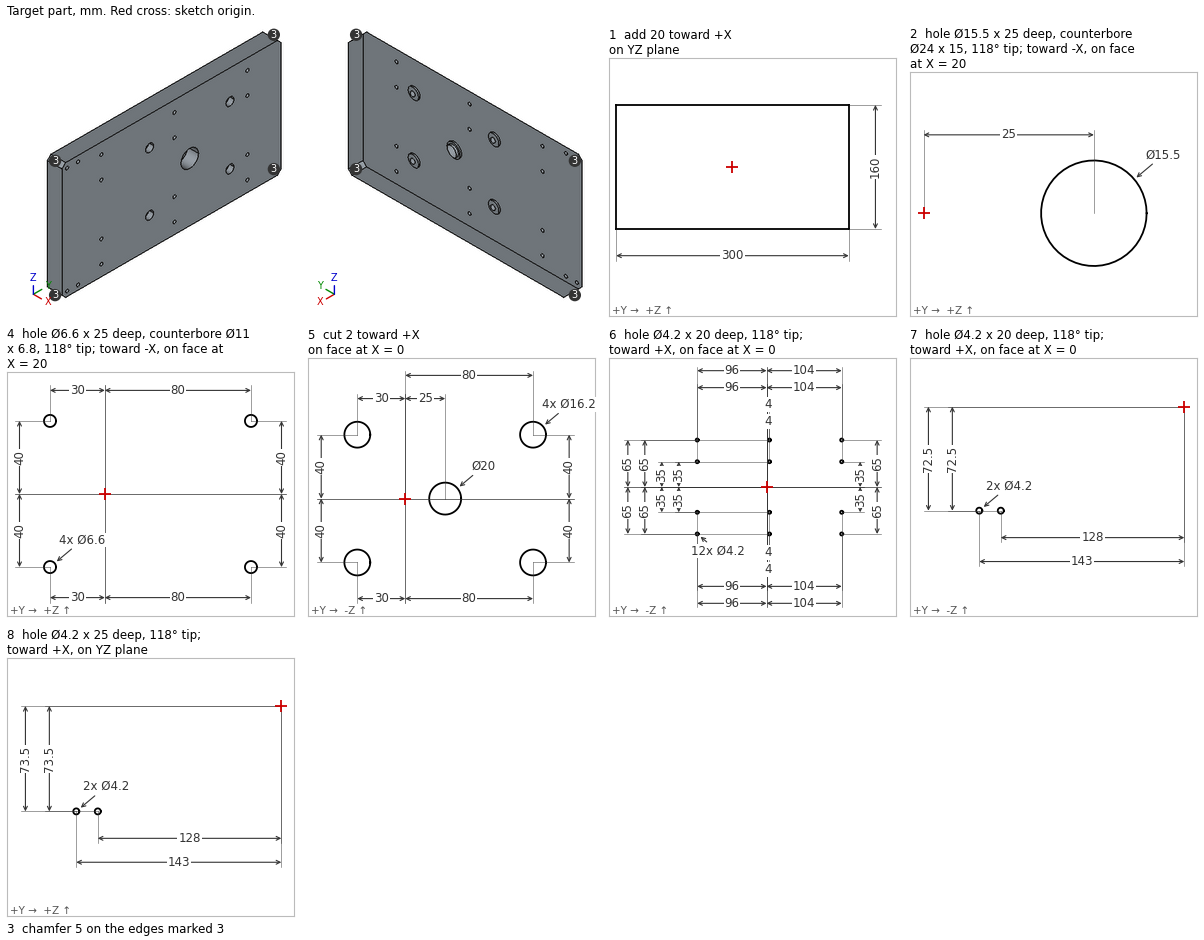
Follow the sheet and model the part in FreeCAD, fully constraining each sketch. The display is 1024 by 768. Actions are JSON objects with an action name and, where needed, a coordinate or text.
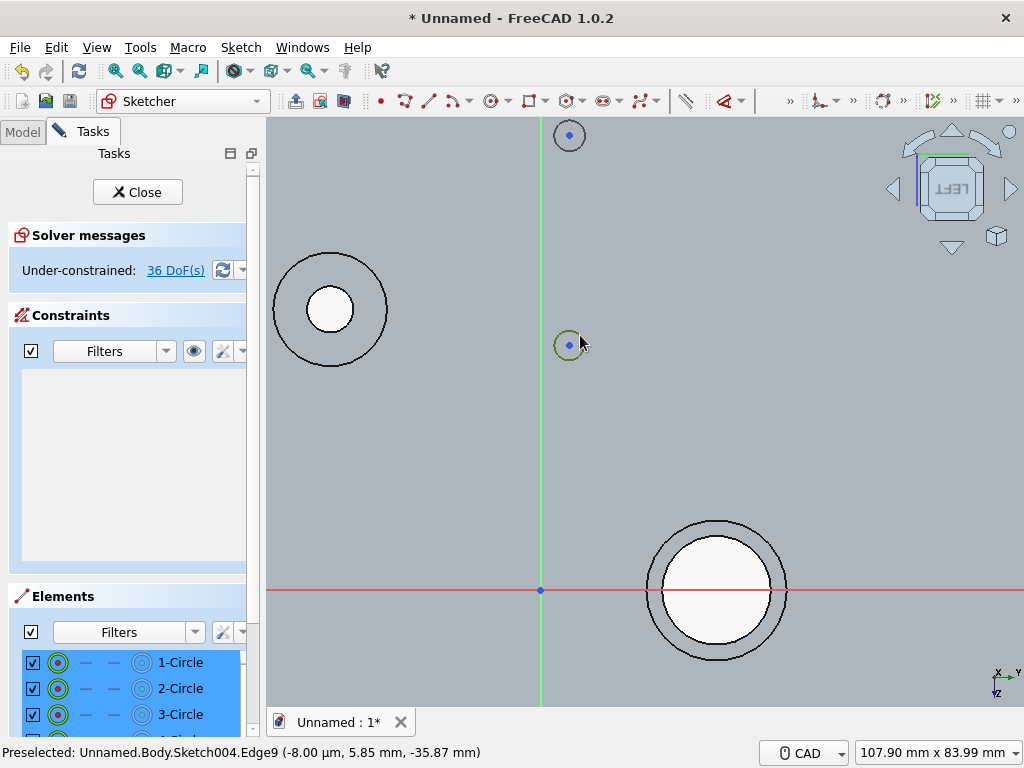
{"action": "left_click", "coordinate": [559, 147]}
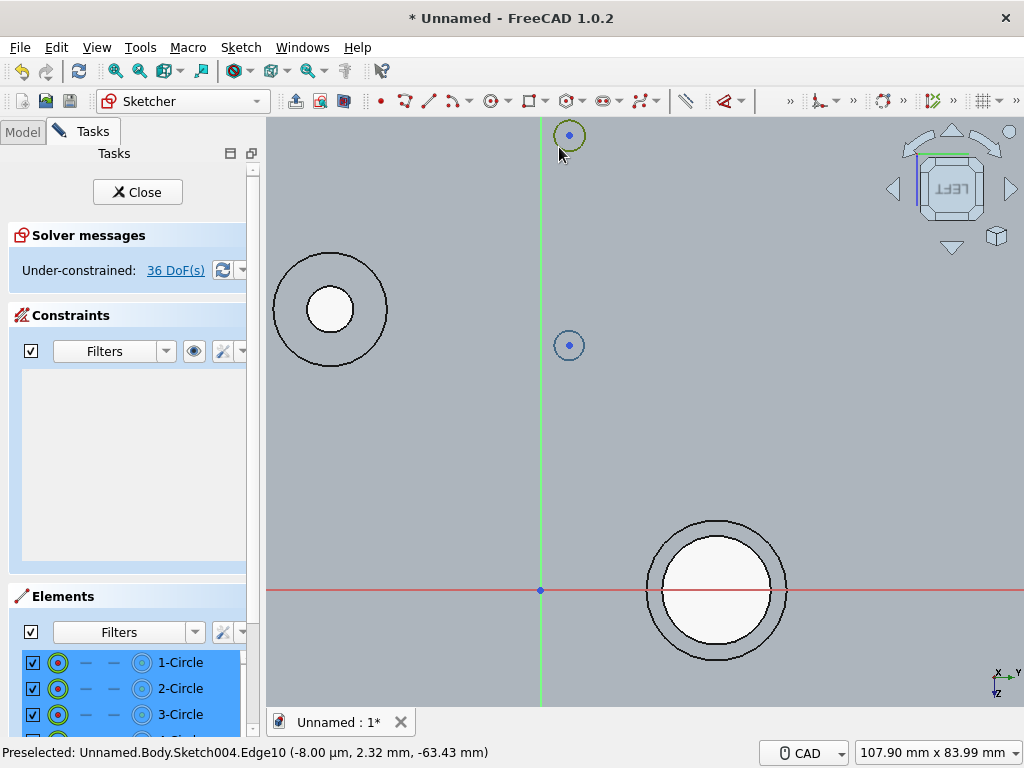
{"action": "scroll", "coordinate": [580, 335], "scroll_direction": "down", "scroll_amount": 6}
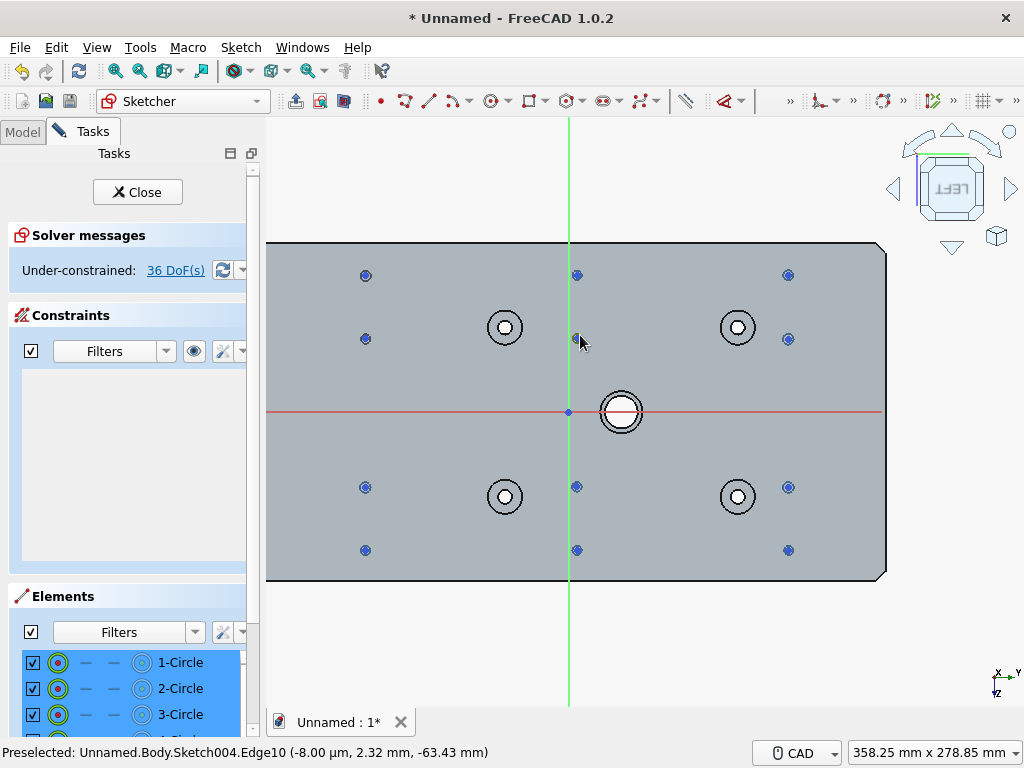
{"action": "scroll", "coordinate": [369, 336], "scroll_direction": "up", "scroll_amount": 6}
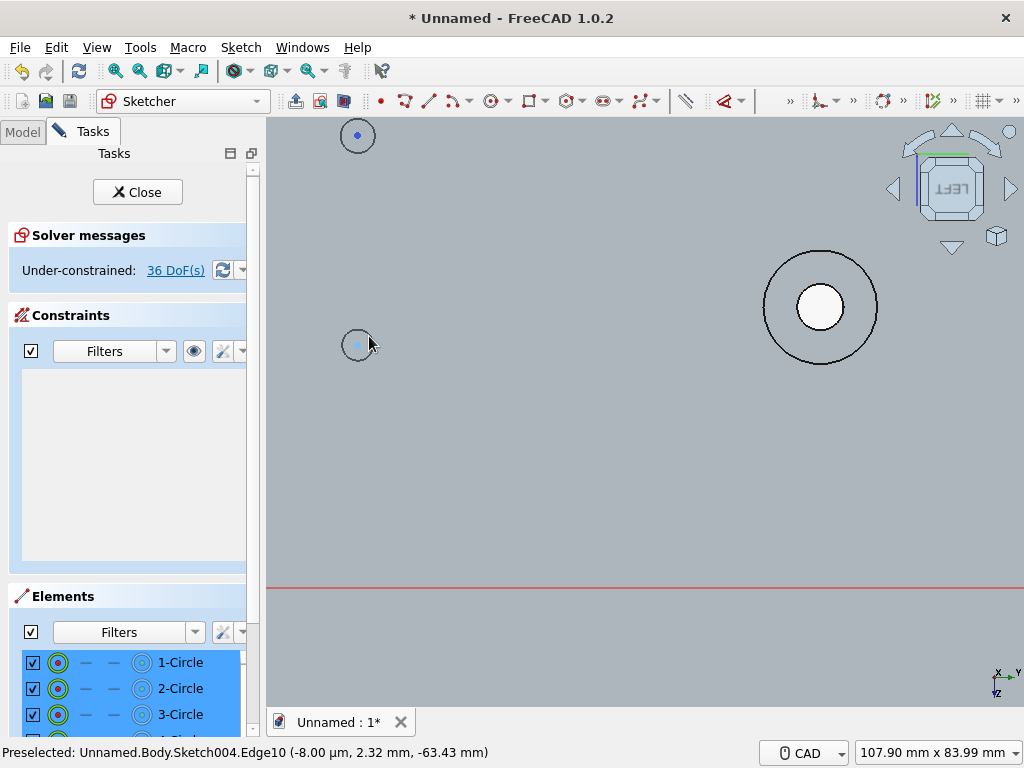
{"action": "left_click", "coordinate": [369, 334]}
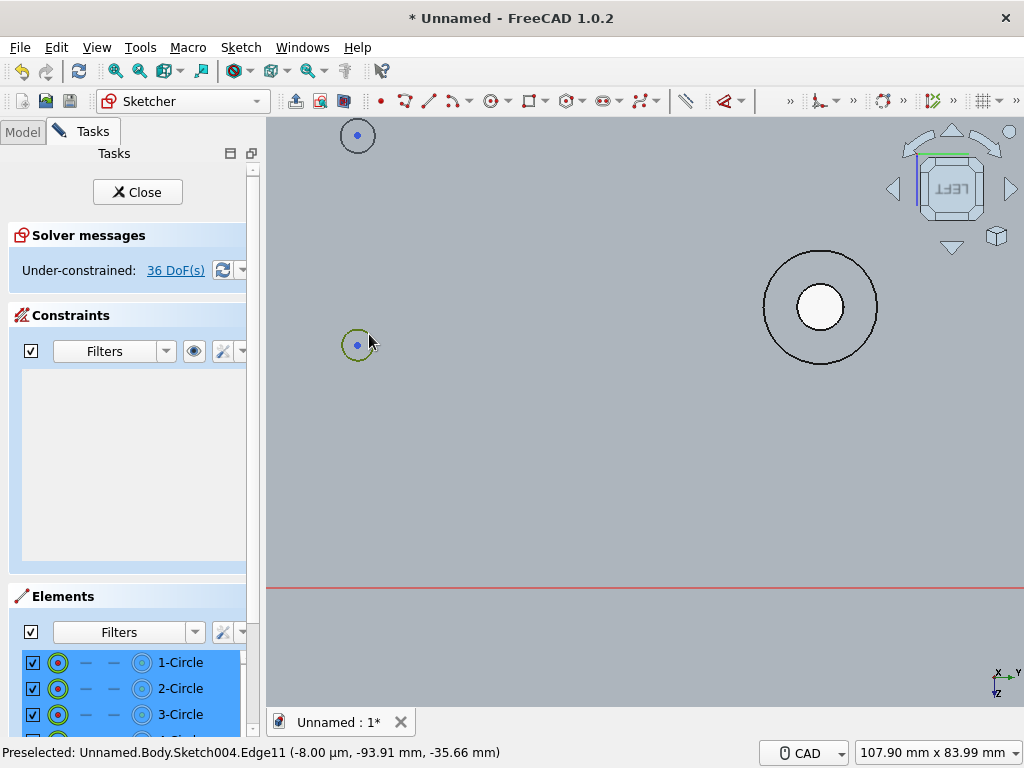
{"action": "left_click", "coordinate": [346, 148]}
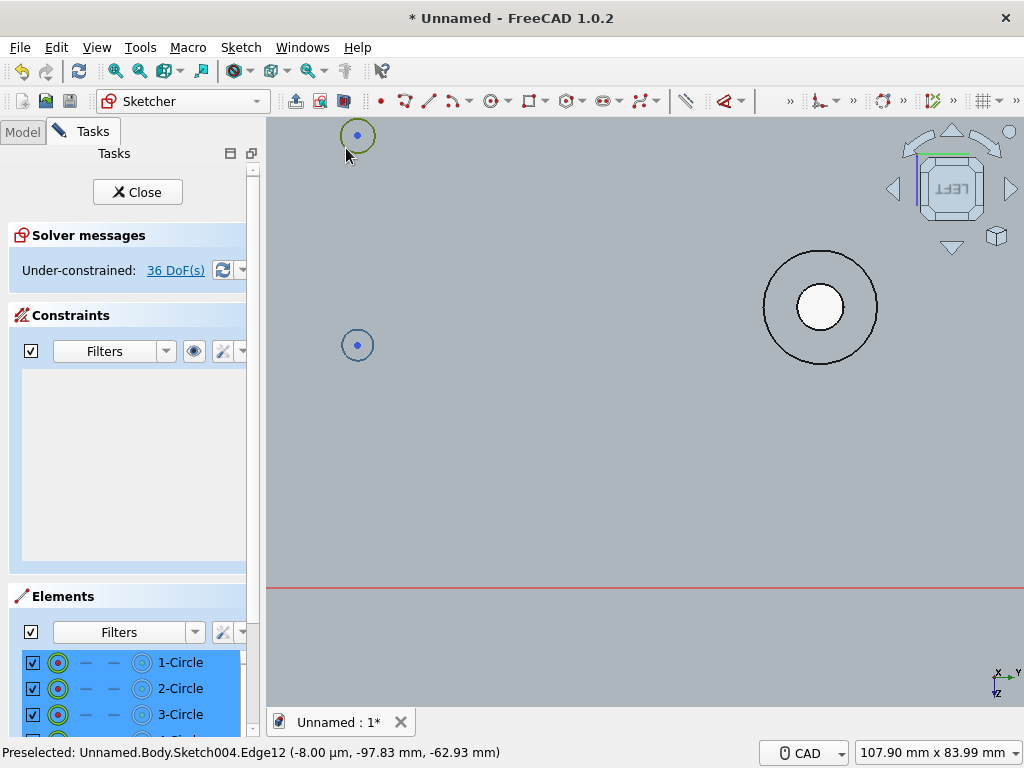
{"action": "key", "text": "e"}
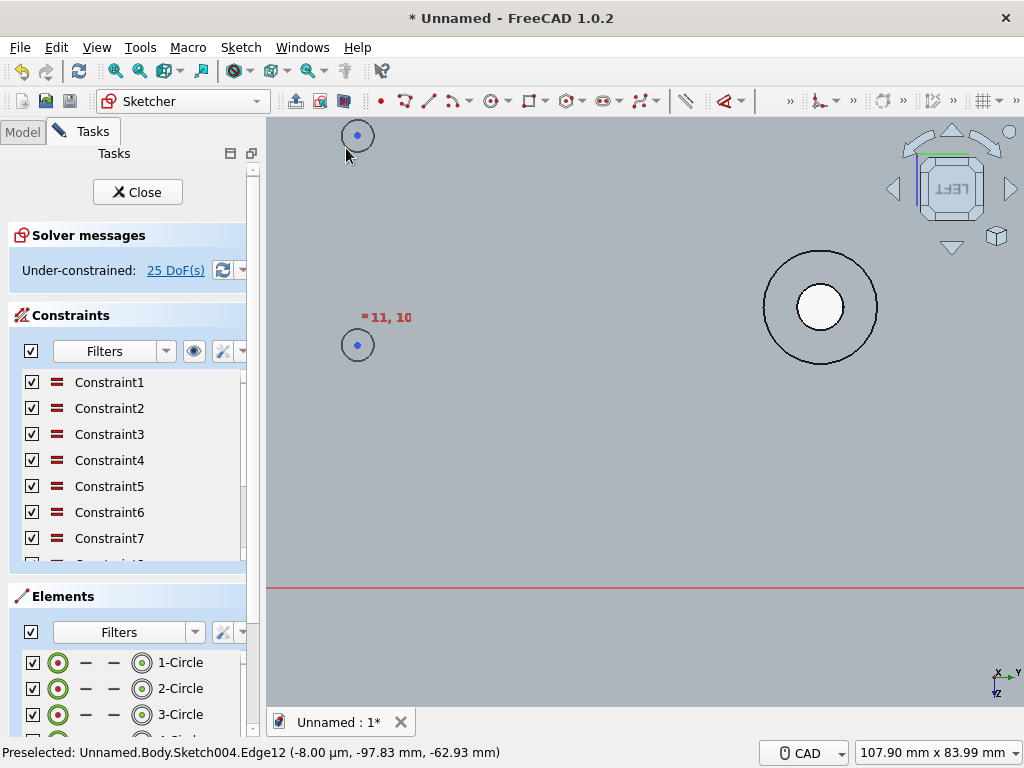
{"action": "key", "text": "d"}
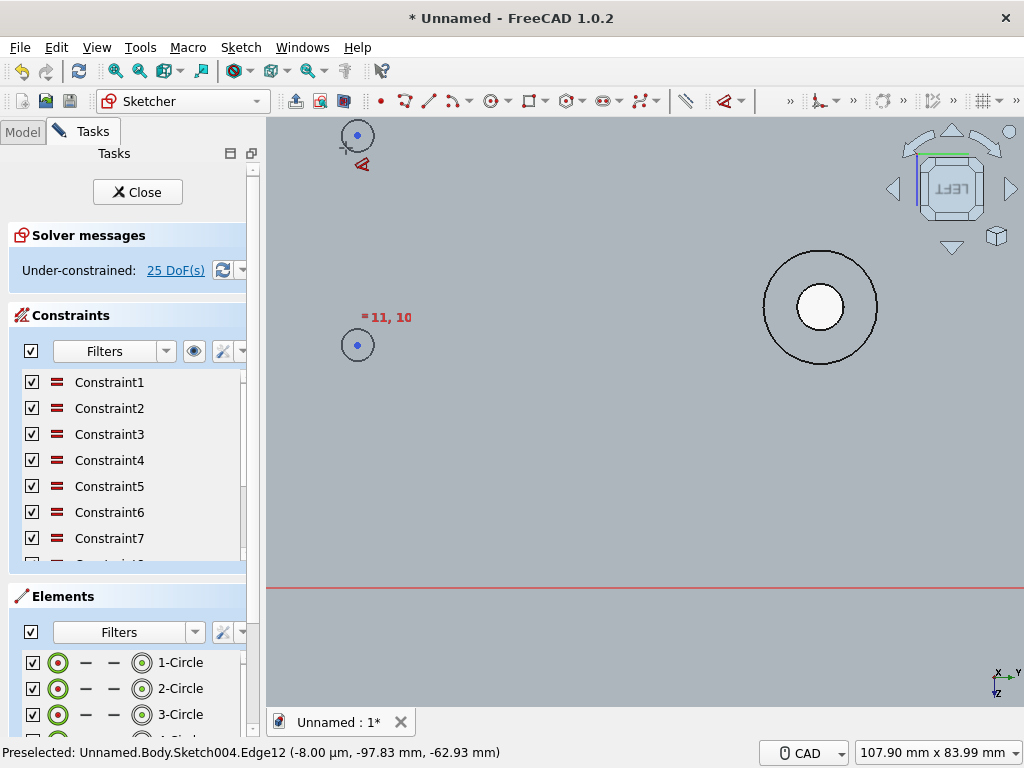
{"action": "scroll", "coordinate": [368, 336], "scroll_direction": "down", "scroll_amount": 6}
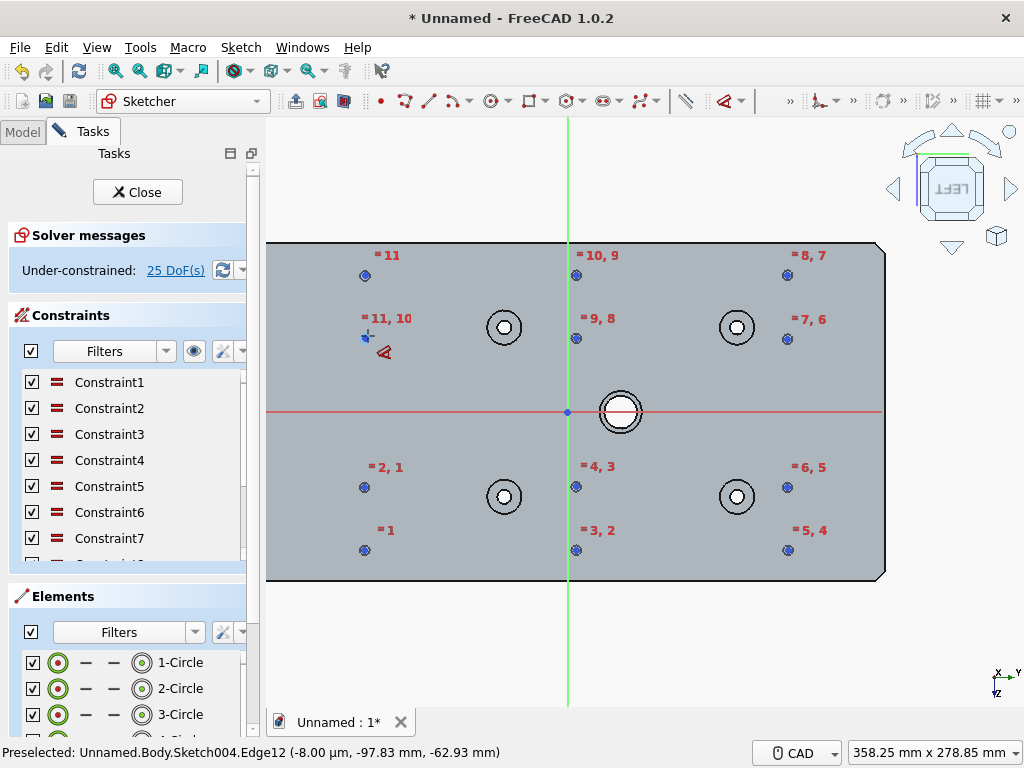
{"action": "scroll", "coordinate": [368, 547], "scroll_direction": "up", "scroll_amount": 8}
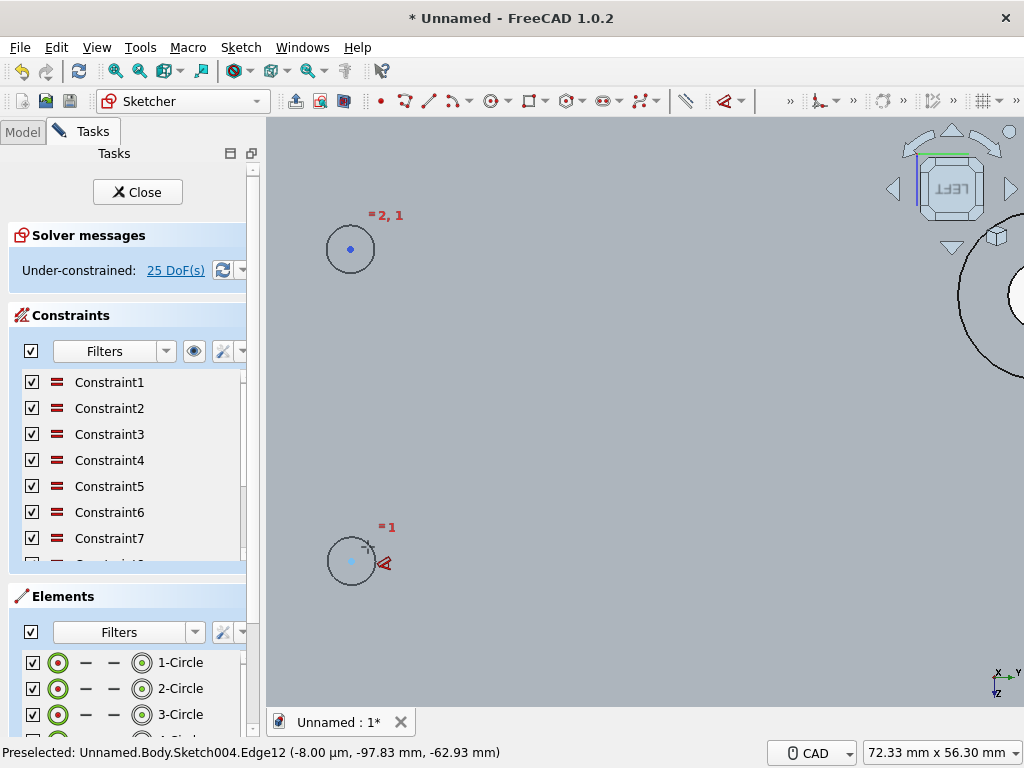
{"action": "left_click", "coordinate": [368, 544]}
{"action": "left_click", "coordinate": [390, 521]}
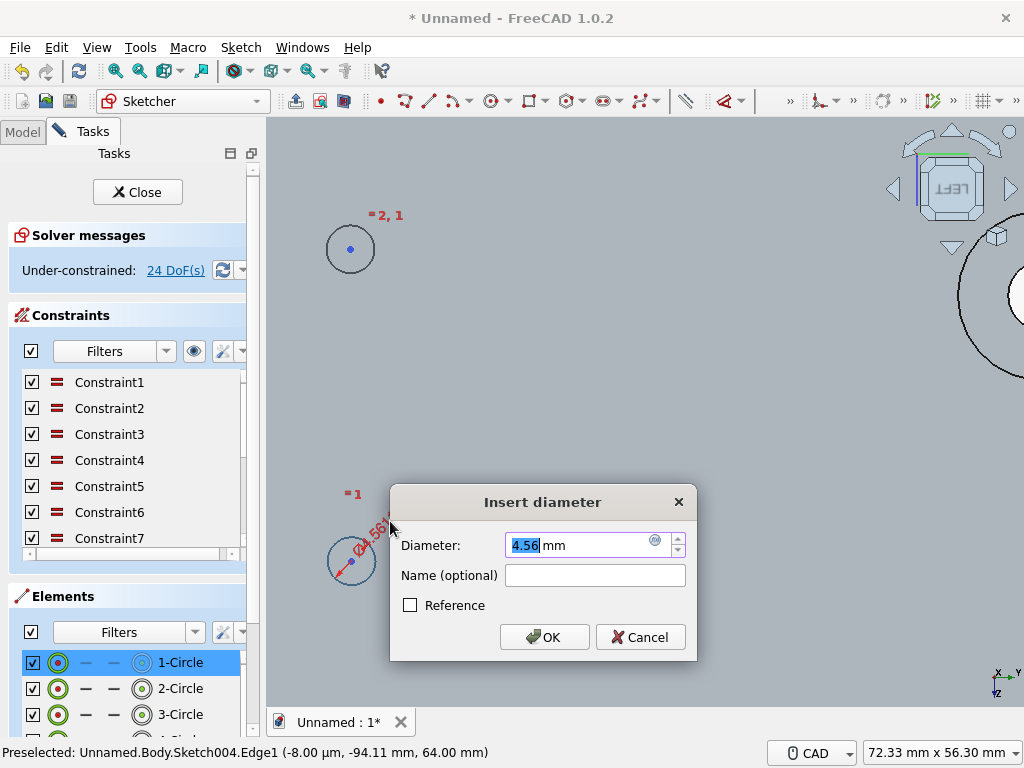
{"action": "type", "text": "4.2"}
{"action": "key", "text": "Return"}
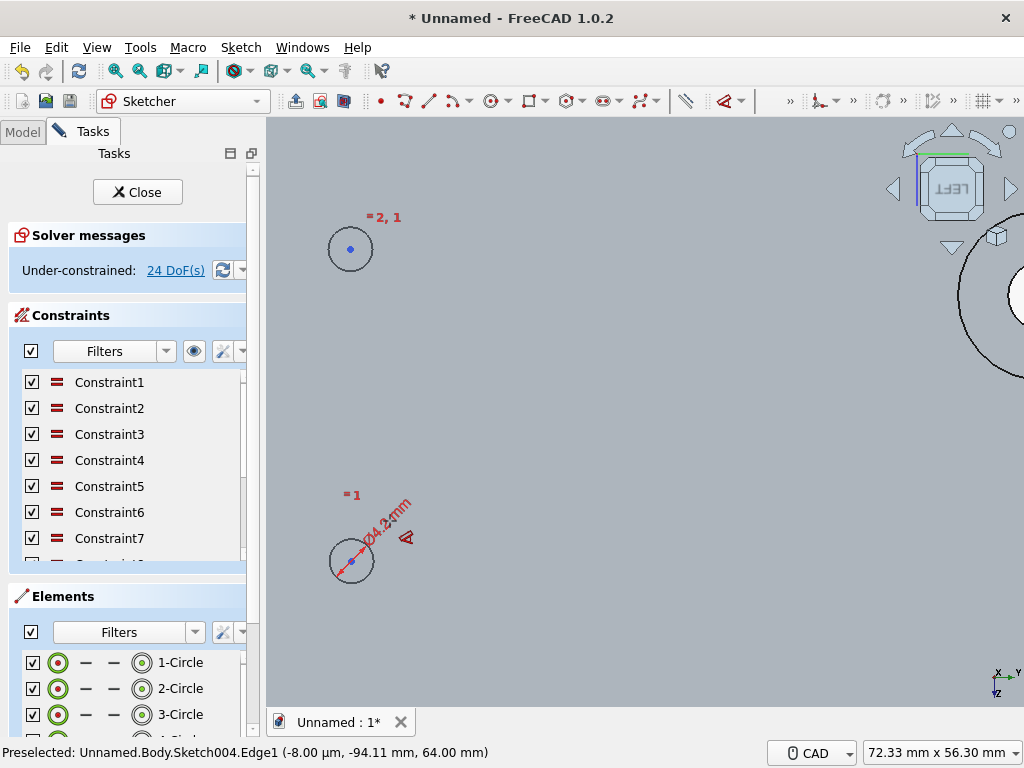
{"action": "scroll", "coordinate": [368, 547], "scroll_direction": "down", "scroll_amount": 8}